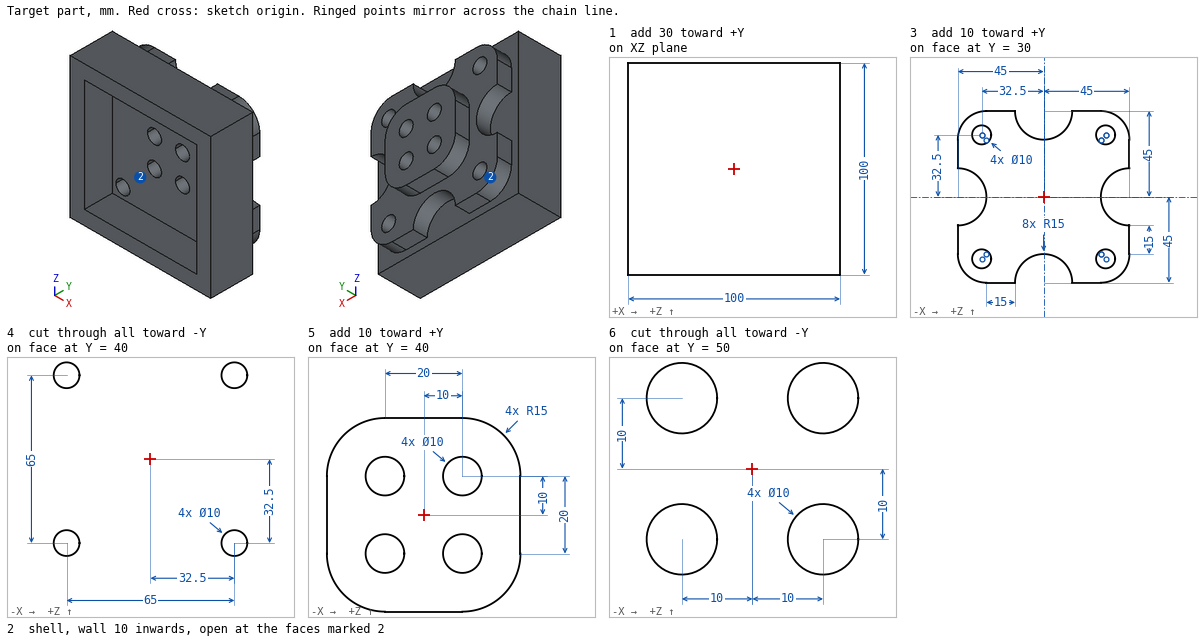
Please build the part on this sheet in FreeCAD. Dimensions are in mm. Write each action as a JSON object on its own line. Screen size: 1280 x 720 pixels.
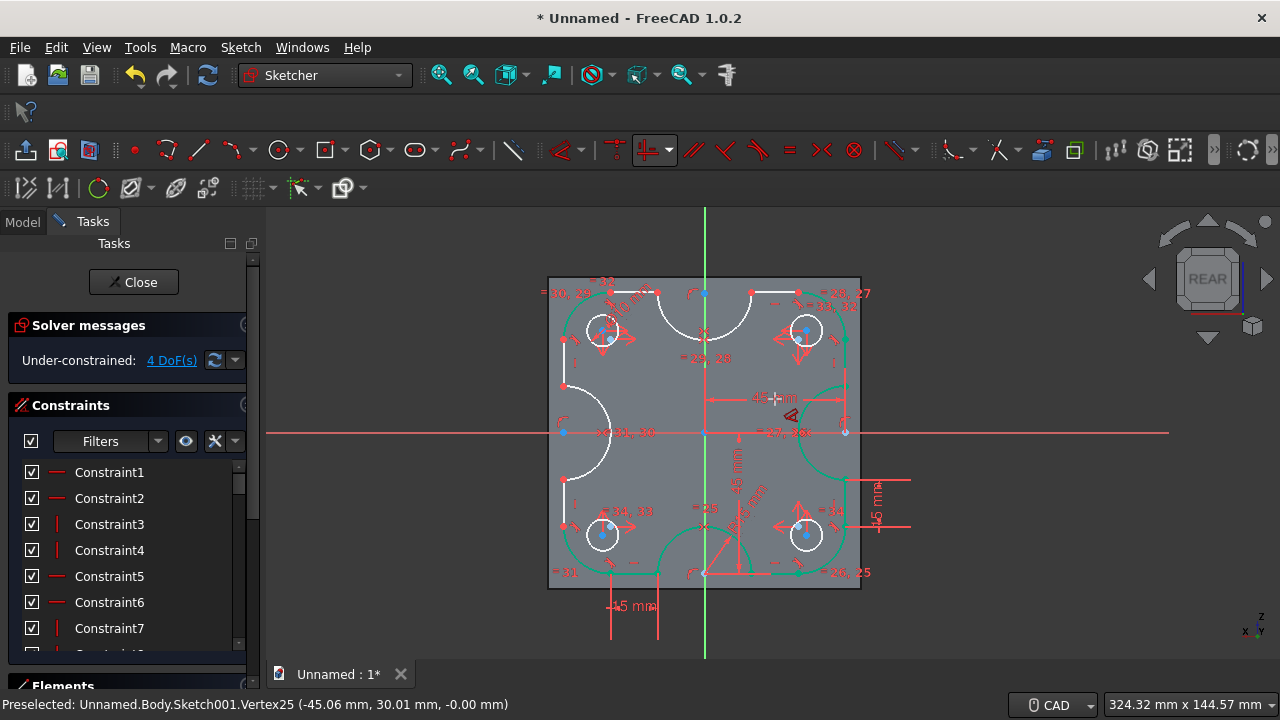
{"action": "left_click", "coordinate": [705, 293]}
{"action": "left_click", "coordinate": [739, 363]}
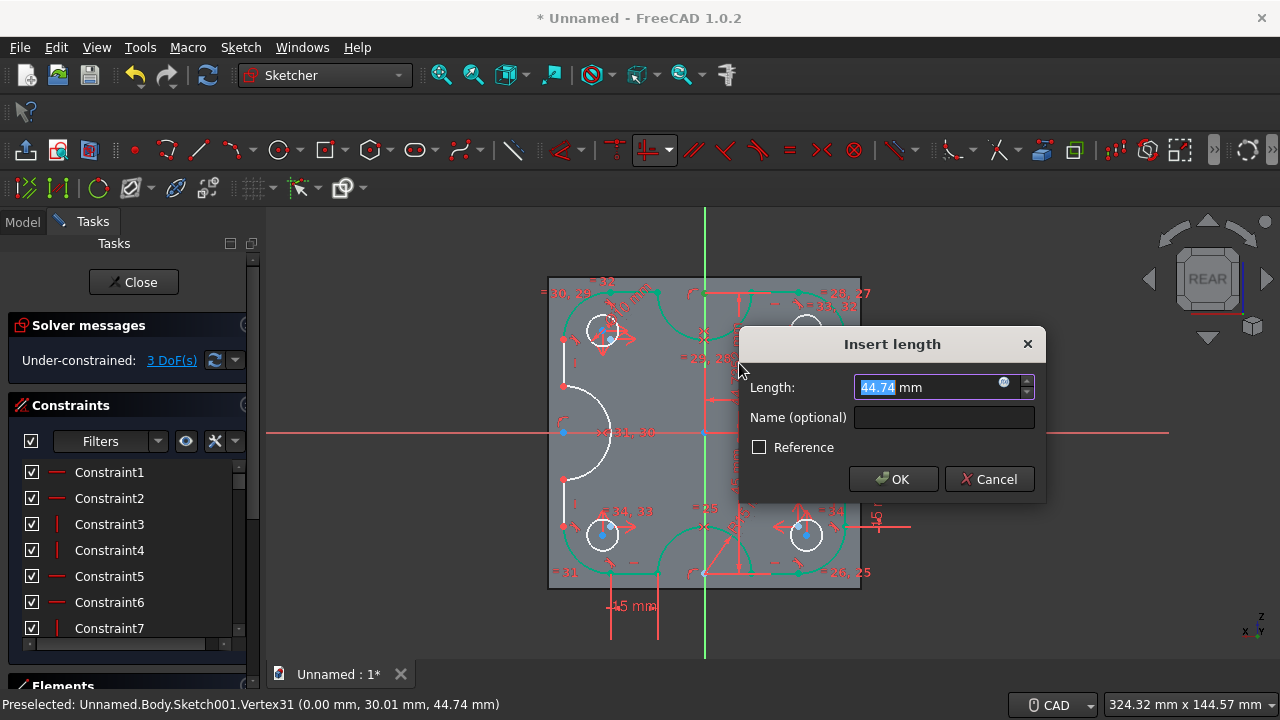
{"action": "type", "text": "45"}
{"action": "key", "text": "Return"}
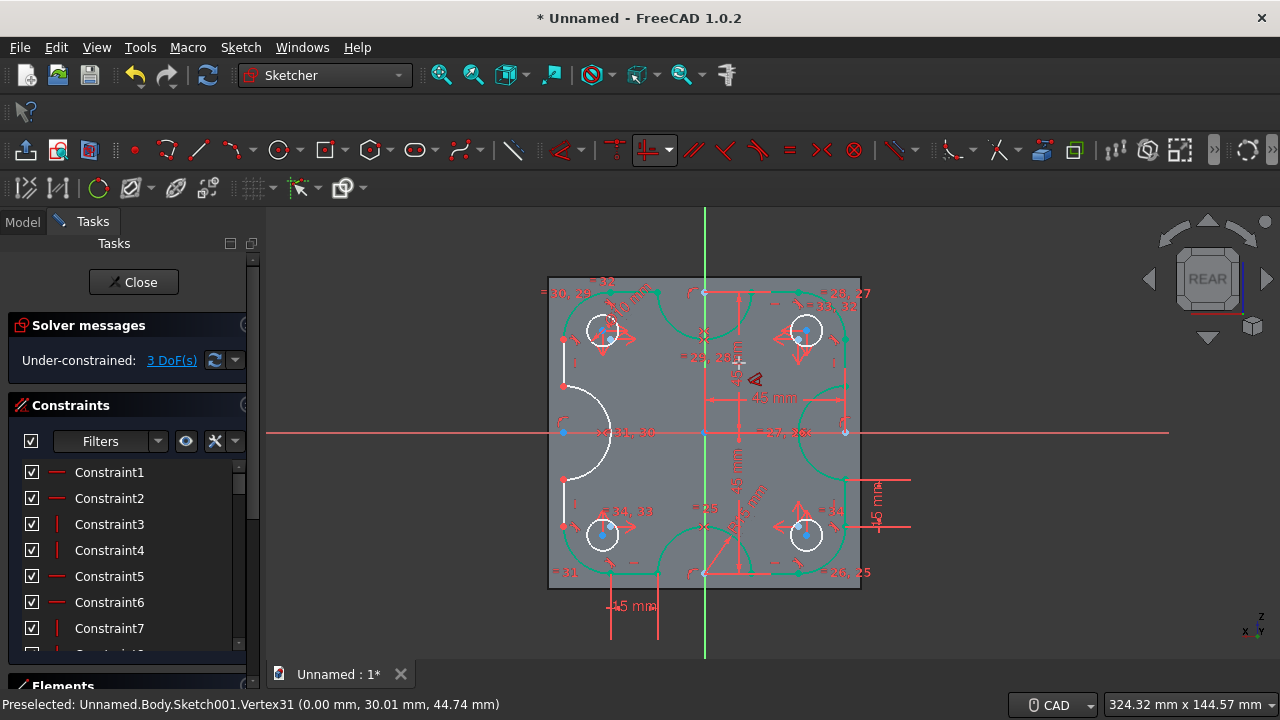
{"action": "left_click", "coordinate": [564, 433]}
{"action": "left_click", "coordinate": [634, 467]}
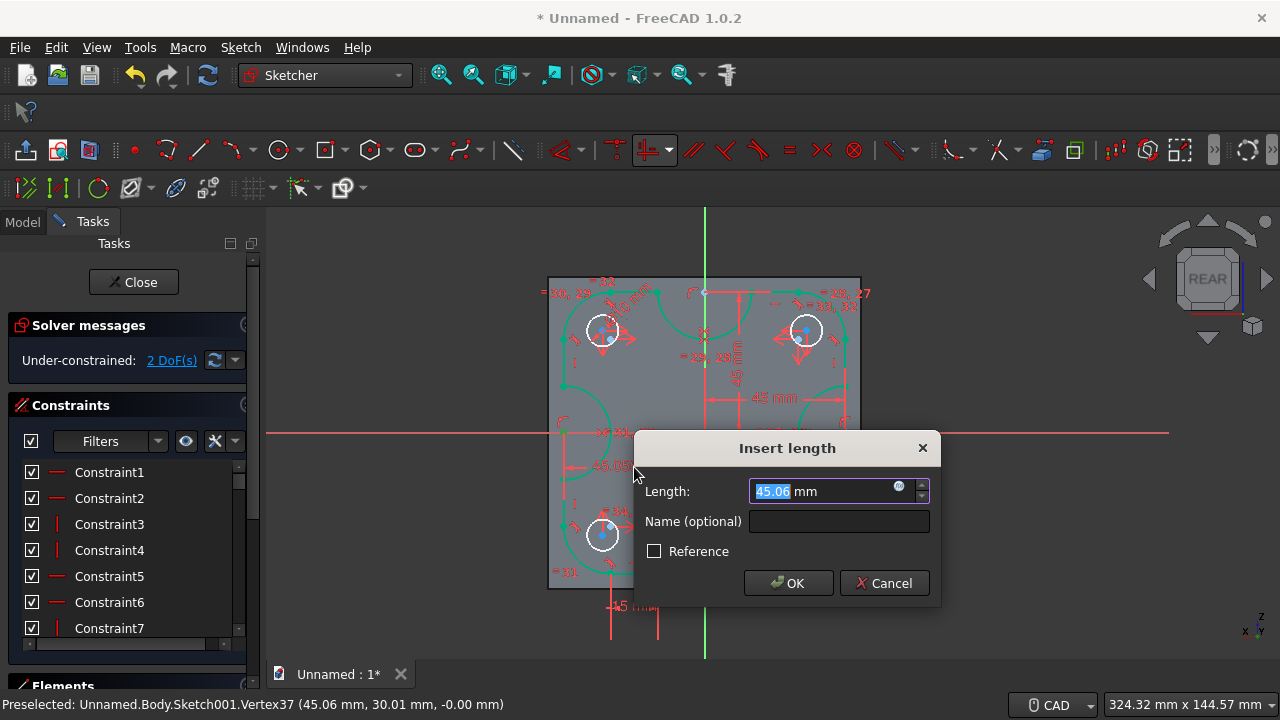
{"action": "type", "text": "45"}
{"action": "key", "text": "Return"}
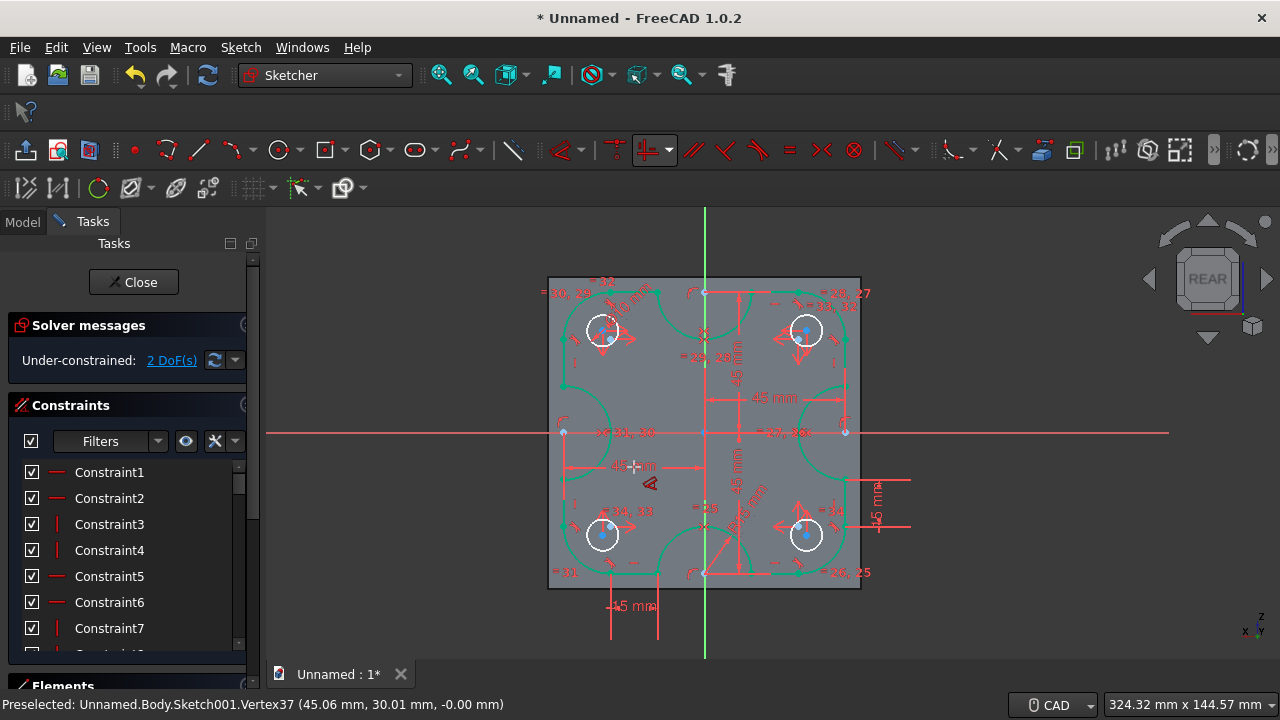
{"action": "left_click", "coordinate": [603, 331]}
{"action": "left_click", "coordinate": [654, 273]}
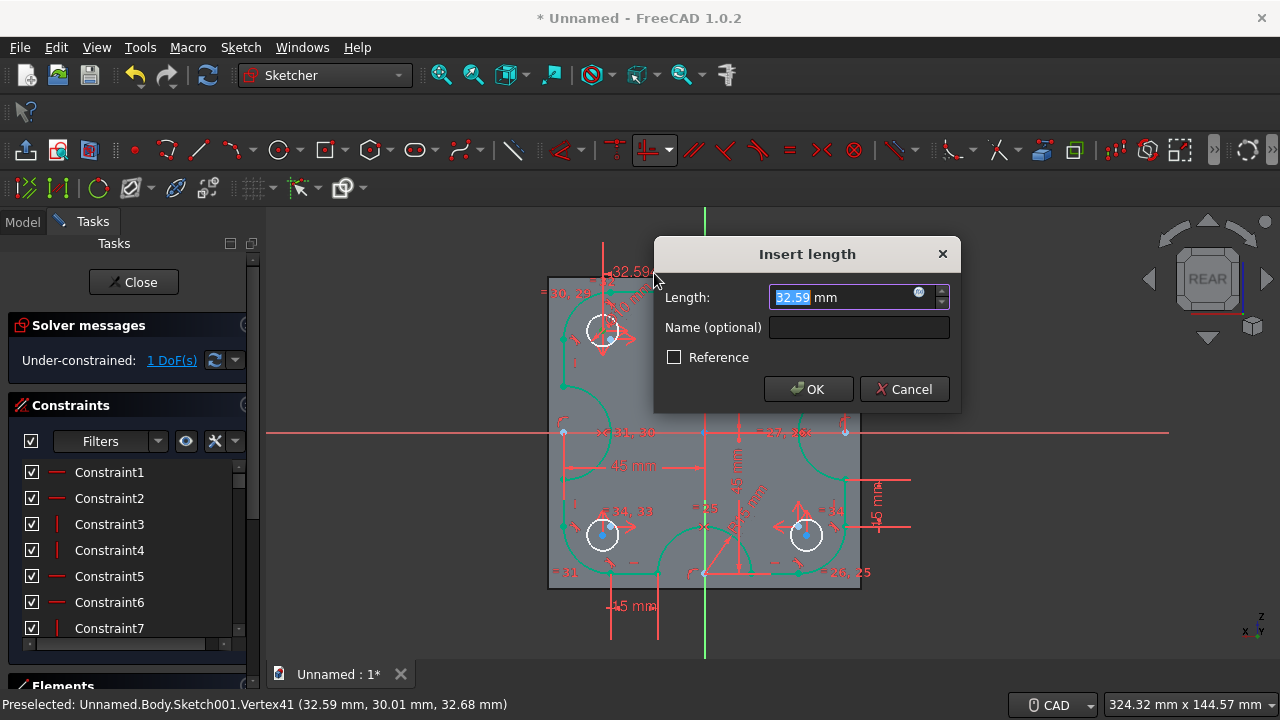
{"action": "type", "text": "32.5"}
{"action": "key", "text": "Return"}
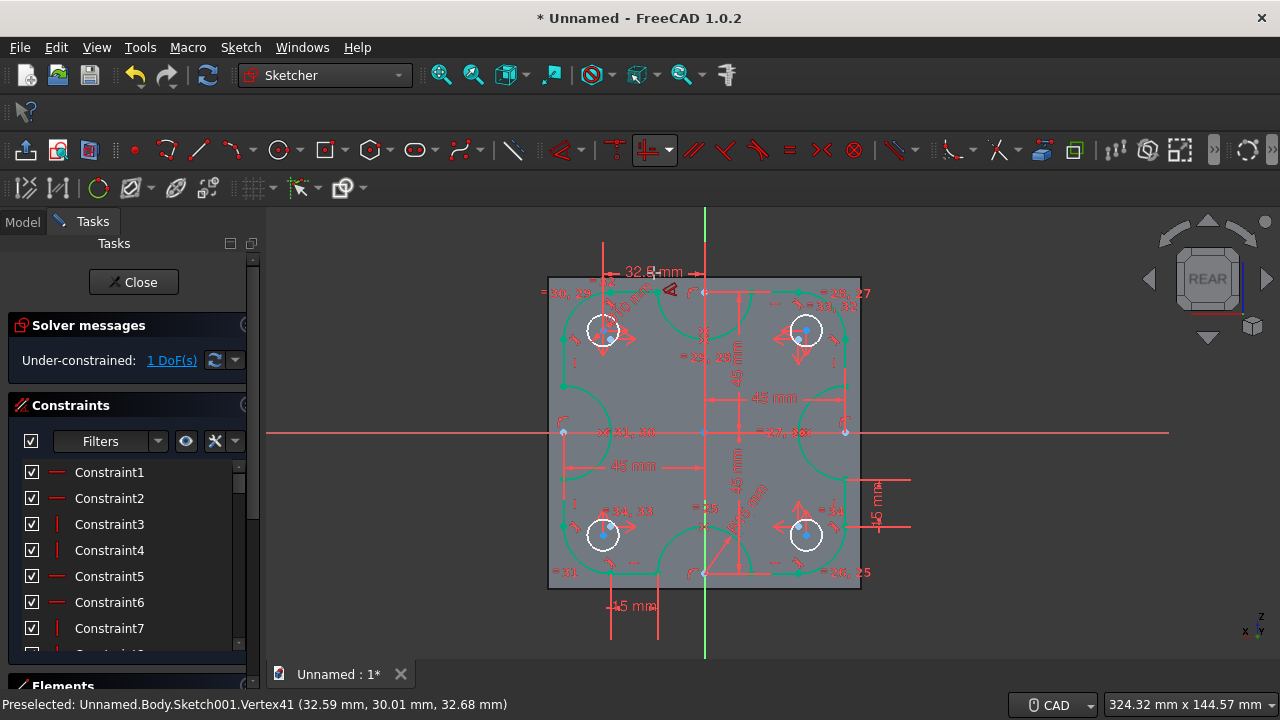
{"action": "left_click", "coordinate": [603, 331]}
{"action": "left_click", "coordinate": [569, 405]}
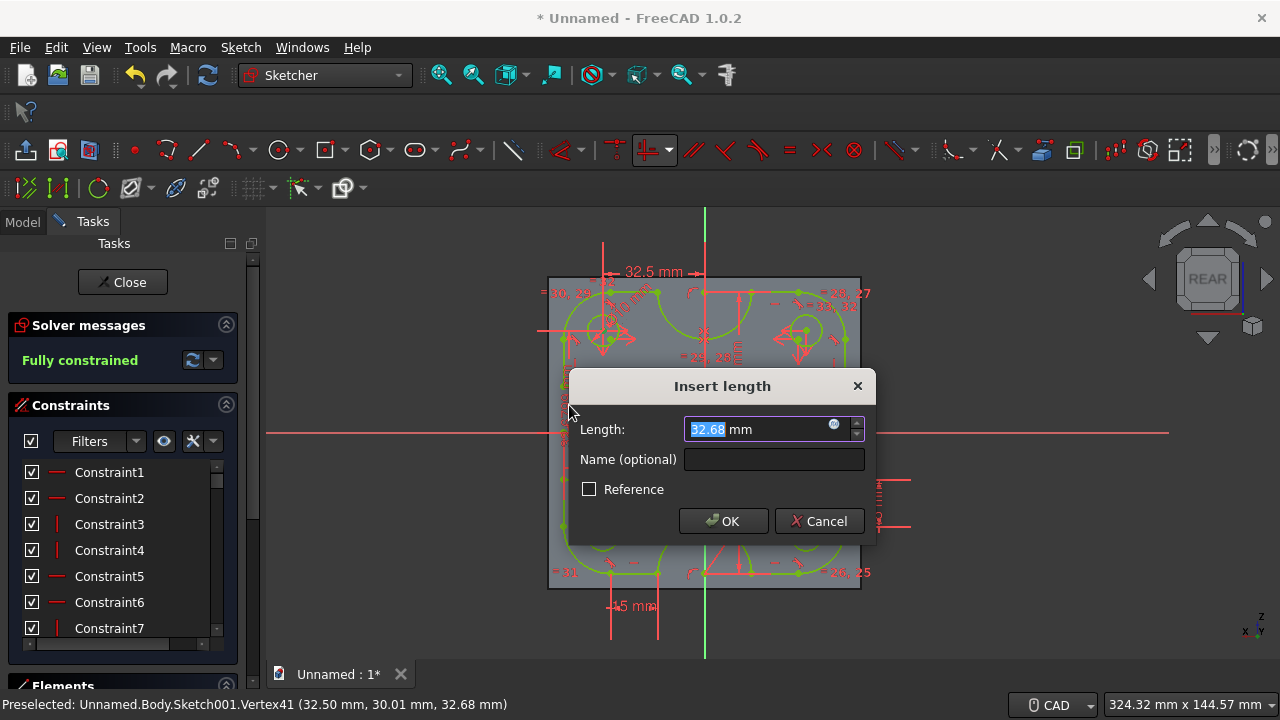
{"action": "type", "text": "32.5"}
{"action": "key", "text": "Return"}
{"action": "key", "text": "Escape"}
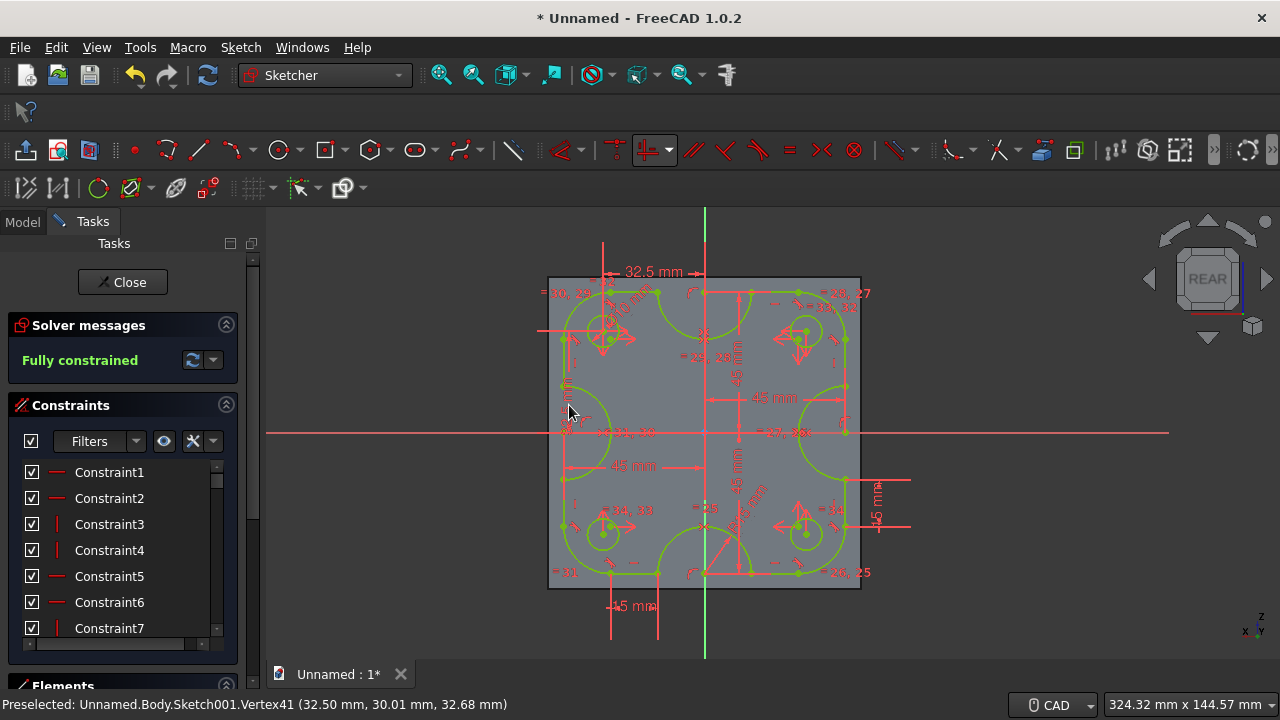
{"action": "left_click", "coordinate": [123, 282]}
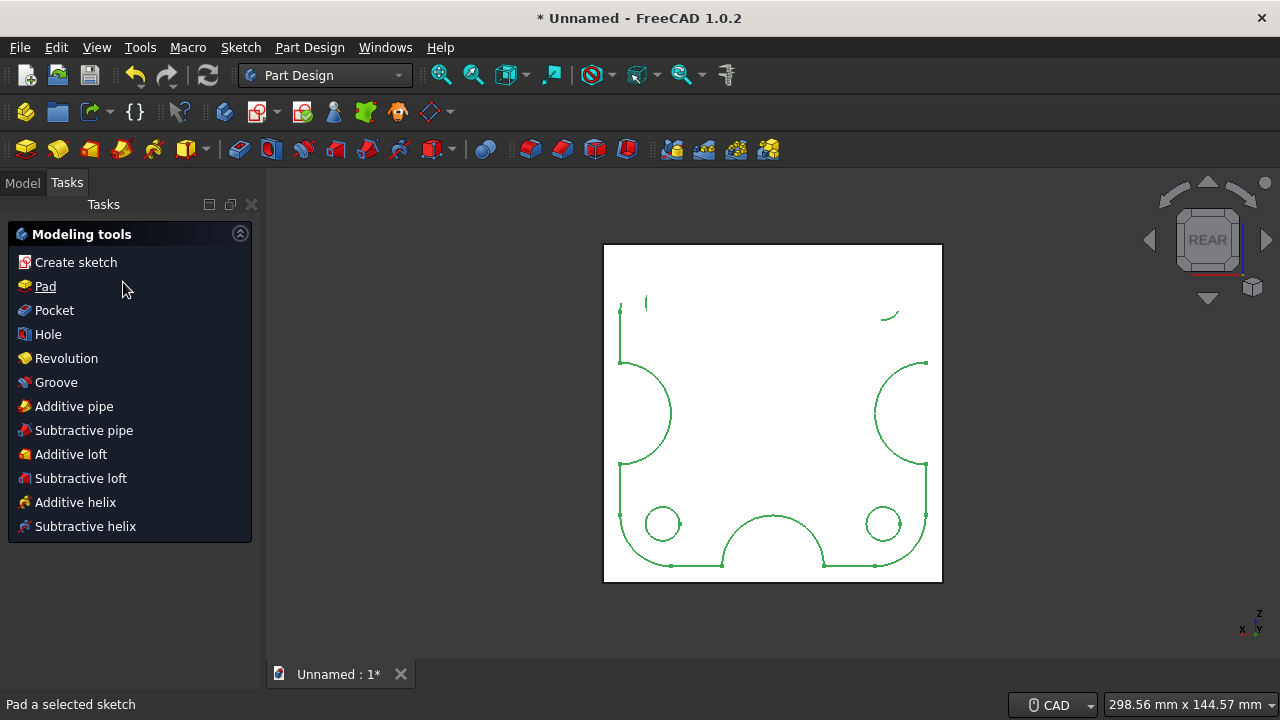
{"action": "left_click", "coordinate": [26, 150]}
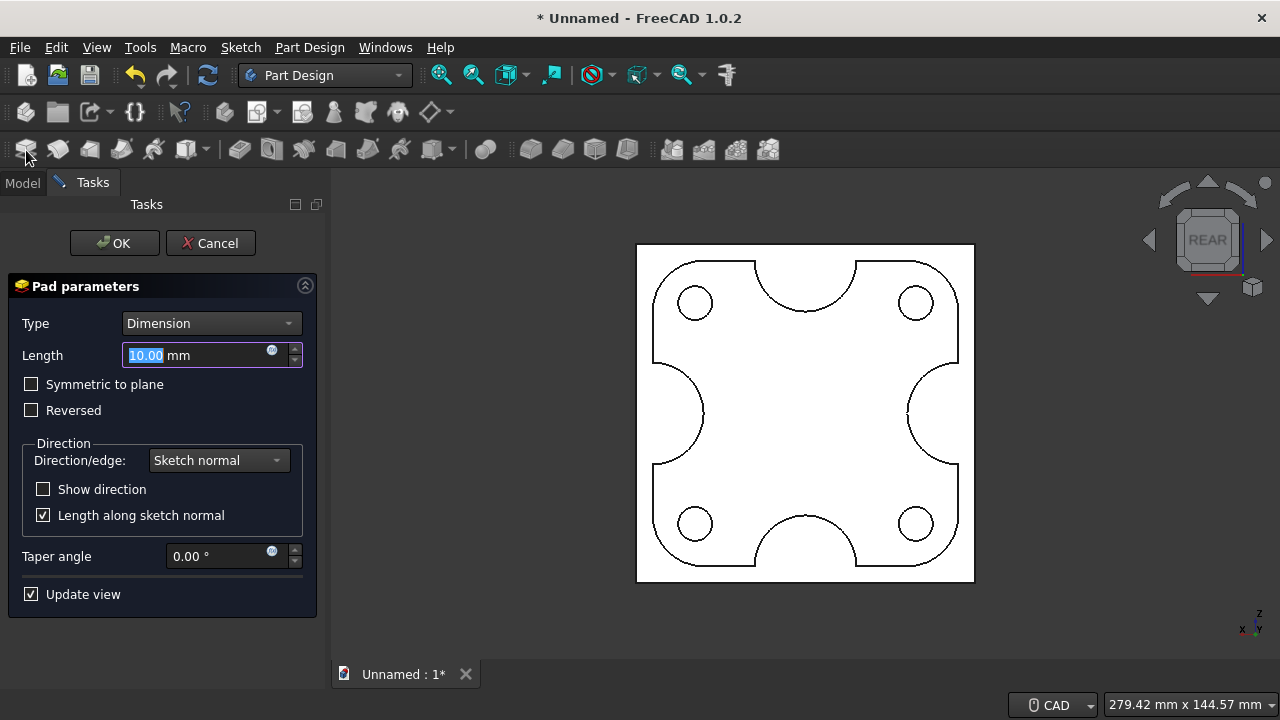
{"action": "type", "text": "10"}
{"action": "key", "text": "Tab"}